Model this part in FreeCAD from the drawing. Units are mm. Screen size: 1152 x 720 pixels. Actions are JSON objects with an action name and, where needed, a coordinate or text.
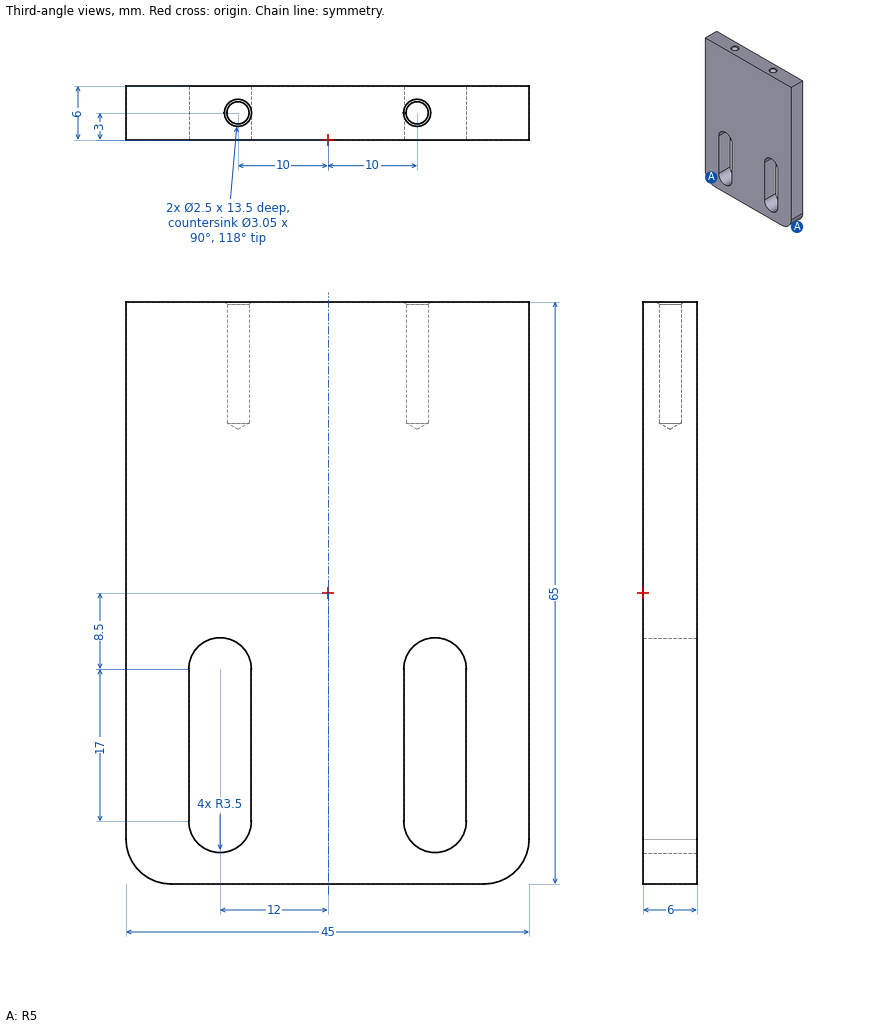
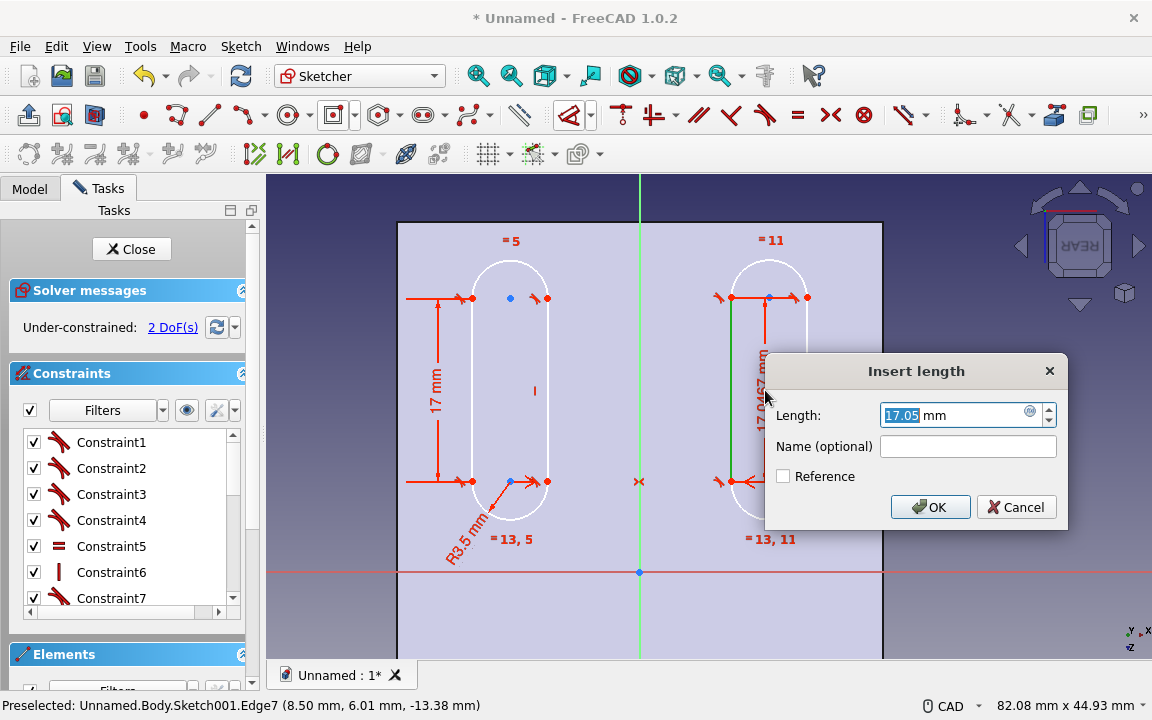
{"action": "type", "text": "17"}
{"action": "key", "text": "Return"}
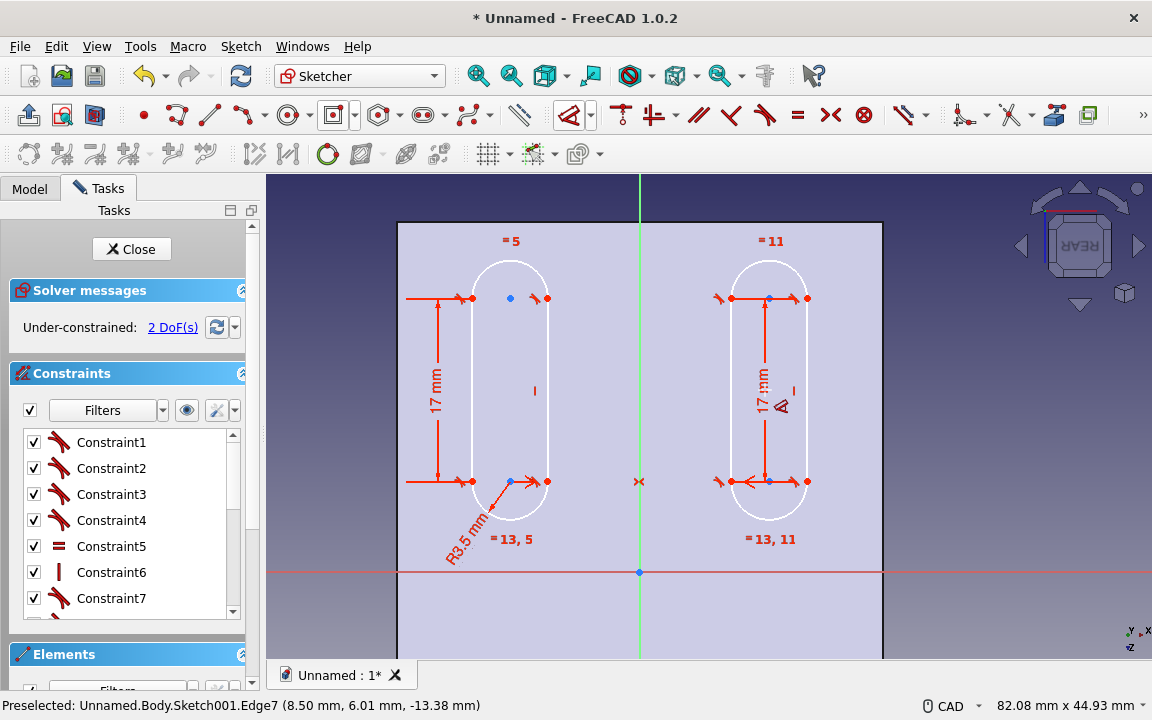
{"action": "left_click", "coordinate": [510, 482]}
{"action": "left_click", "coordinate": [575, 606]}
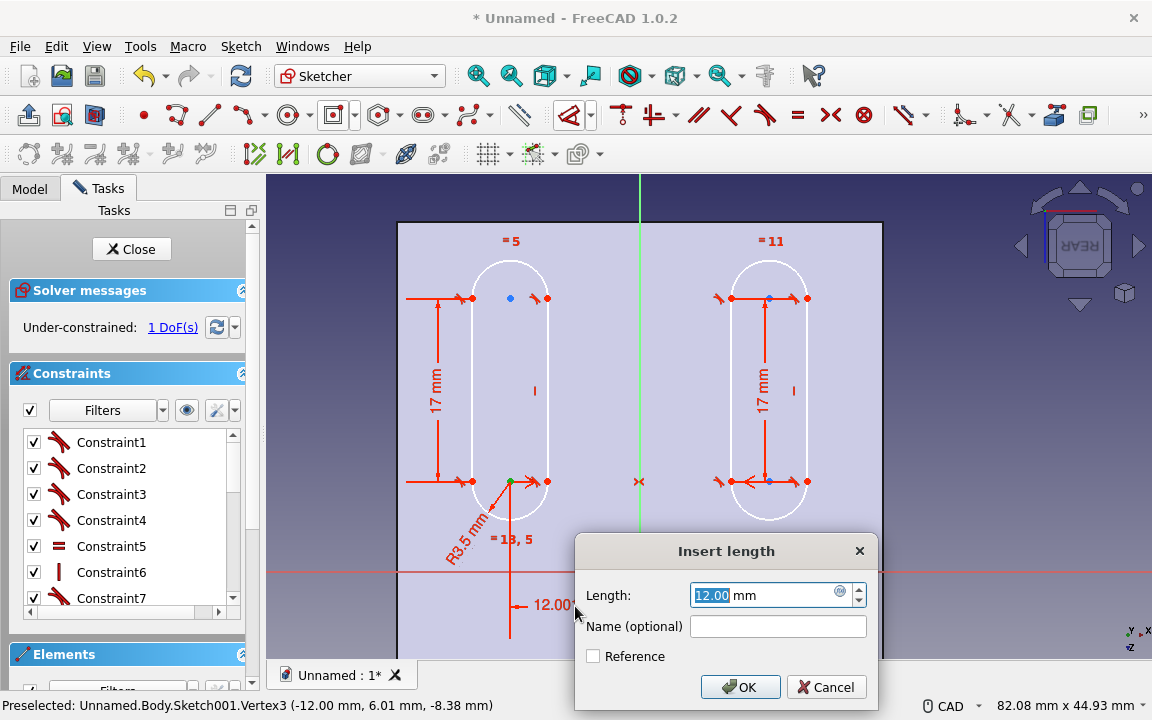
{"action": "type", "text": "12"}
{"action": "key", "text": "Return"}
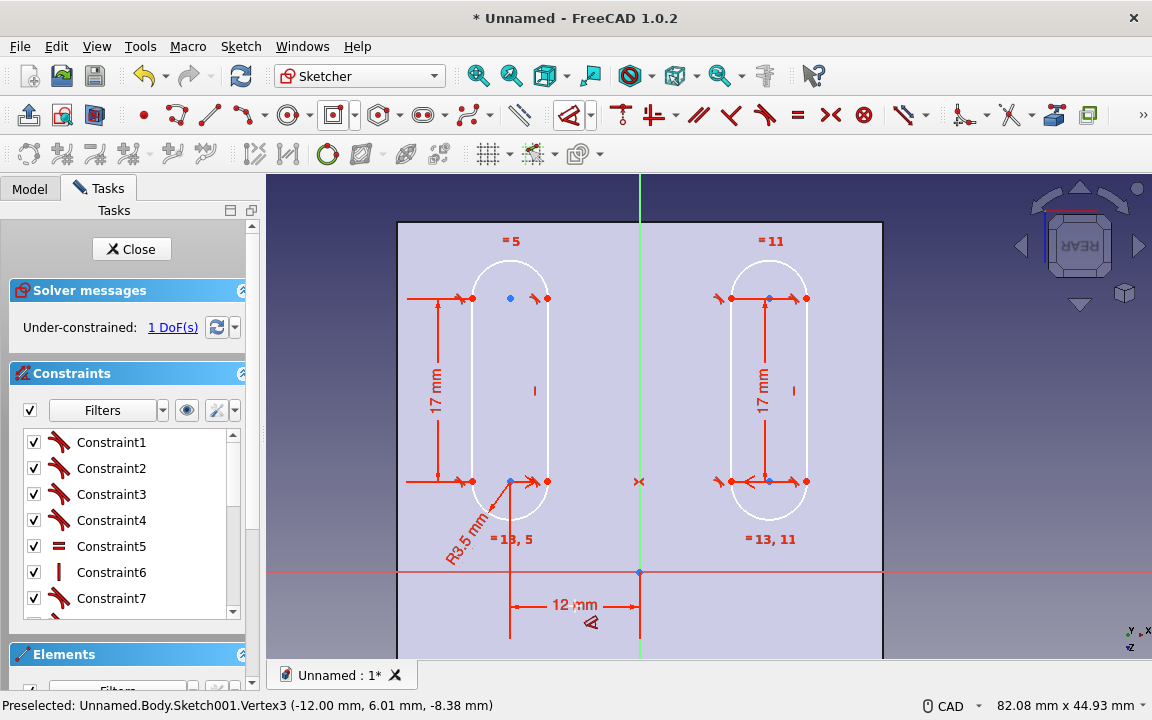
{"action": "left_click", "coordinate": [472, 482]}
{"action": "left_click", "coordinate": [438, 506]}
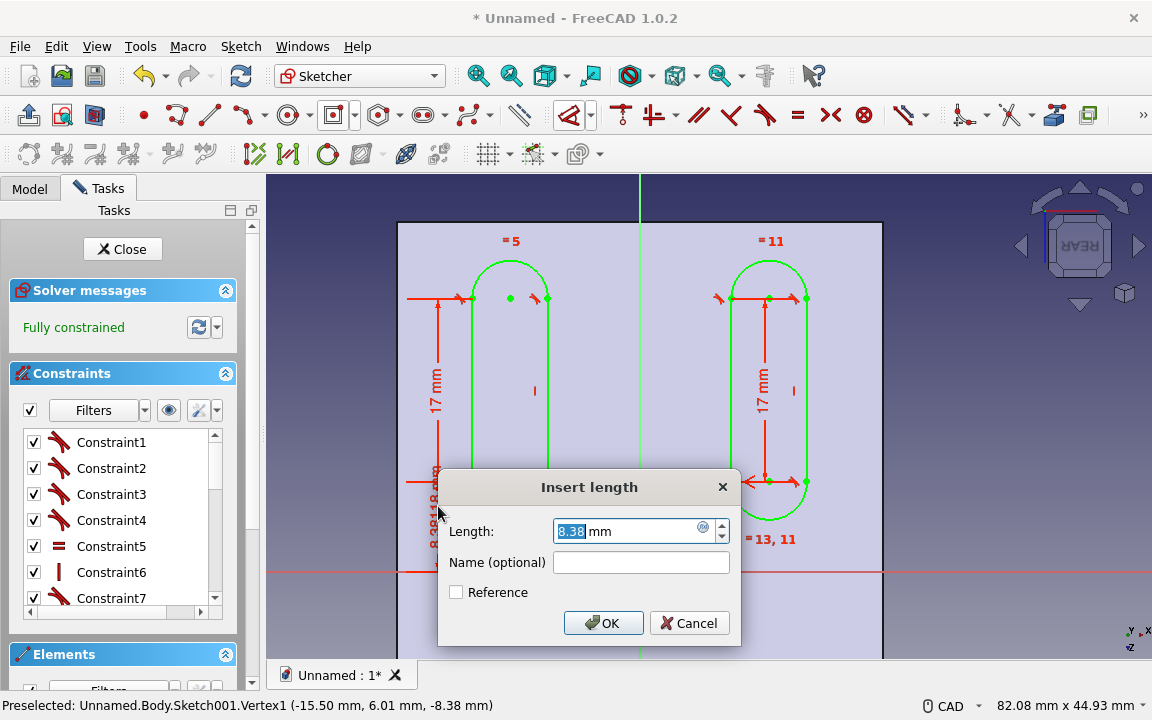
{"action": "type", "text": "8.5"}
{"action": "key", "text": "Return"}
{"action": "key", "text": "Escape"}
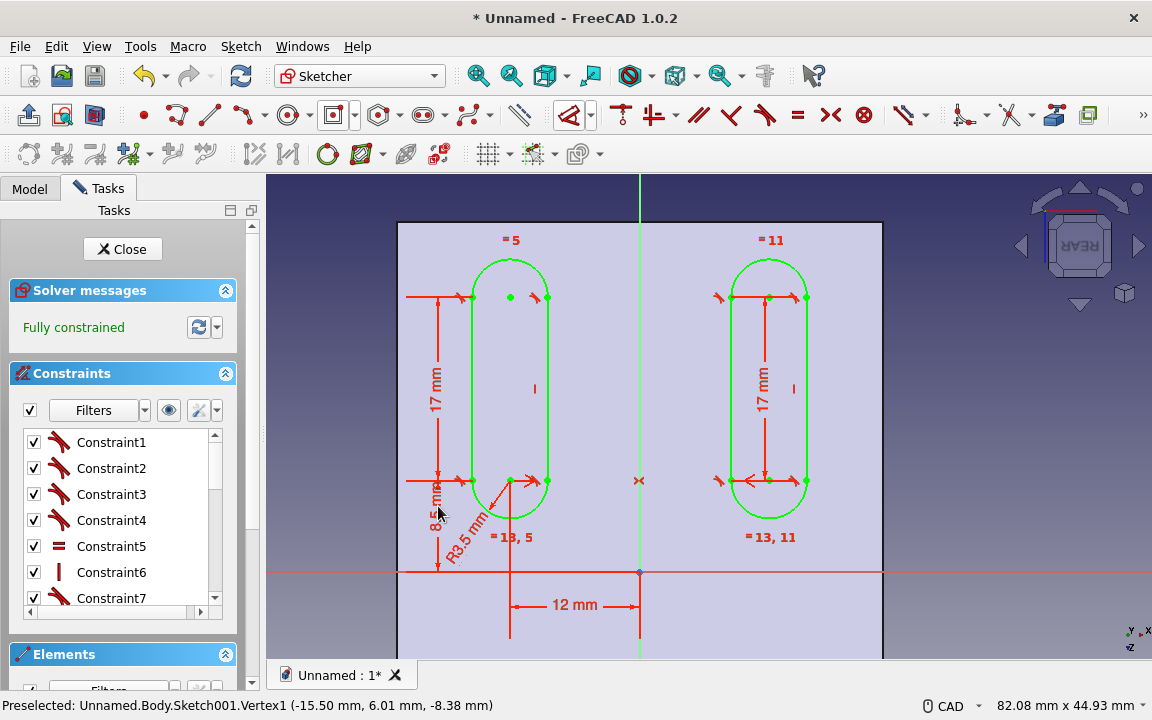
{"action": "left_click", "coordinate": [123, 249]}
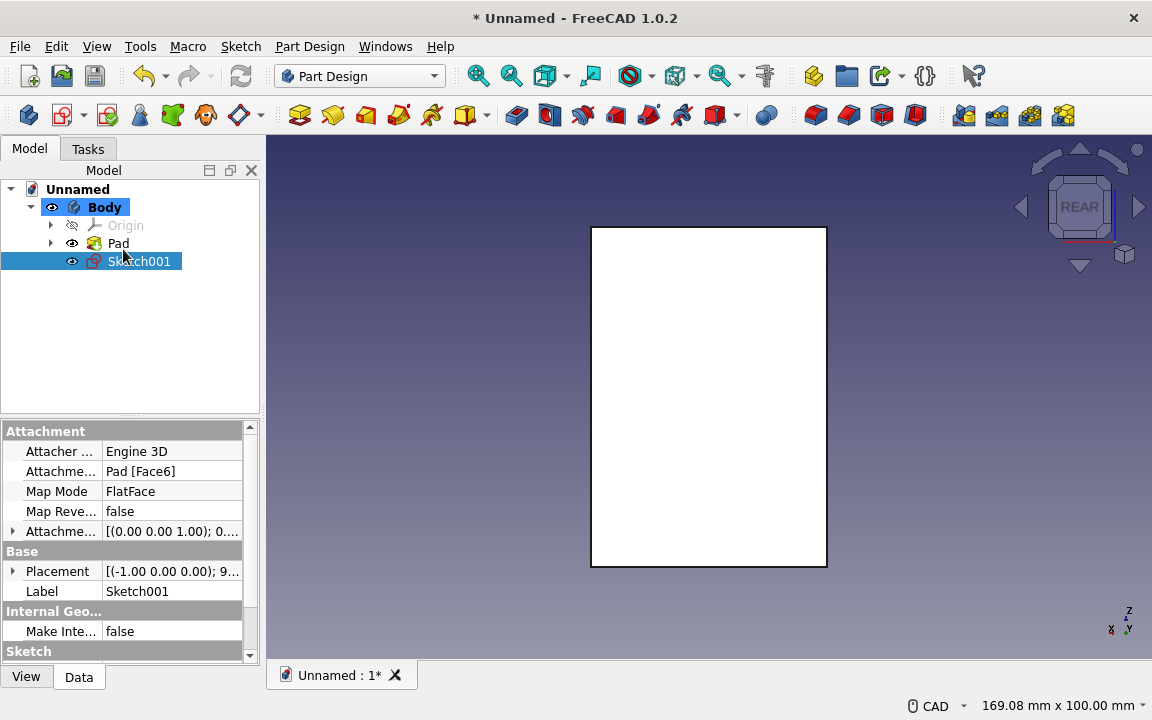
{"action": "left_click", "coordinate": [517, 116]}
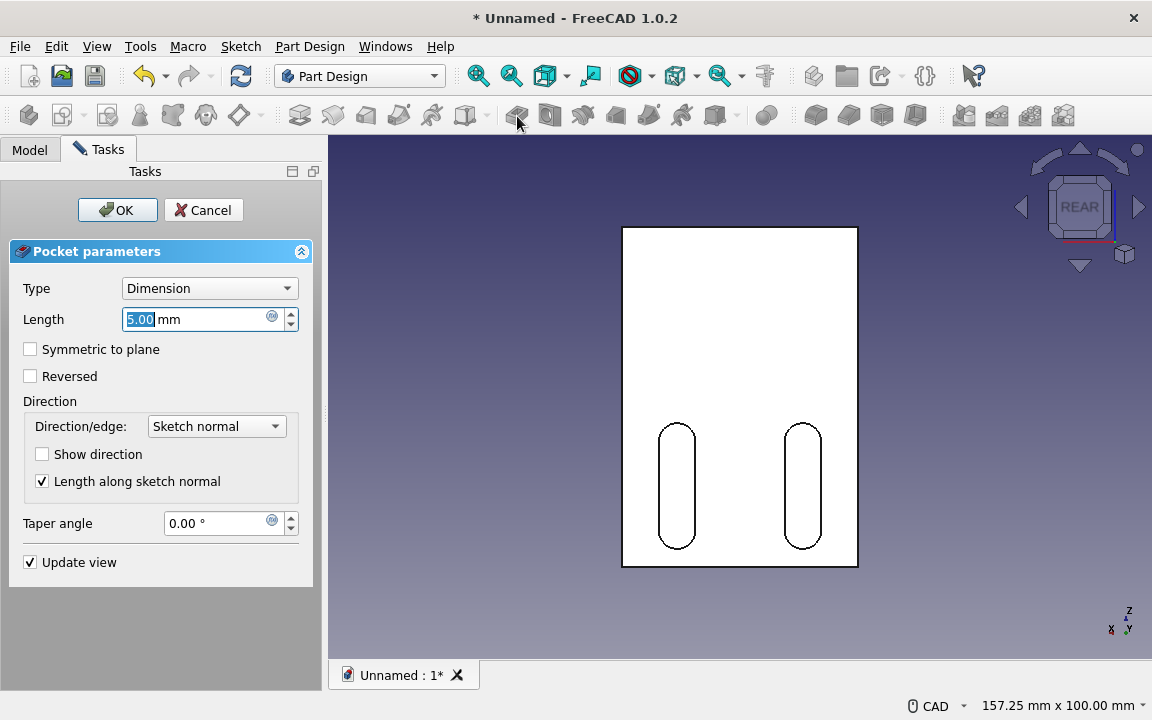
{"action": "type", "text": "6"}
{"action": "key", "text": "Tab"}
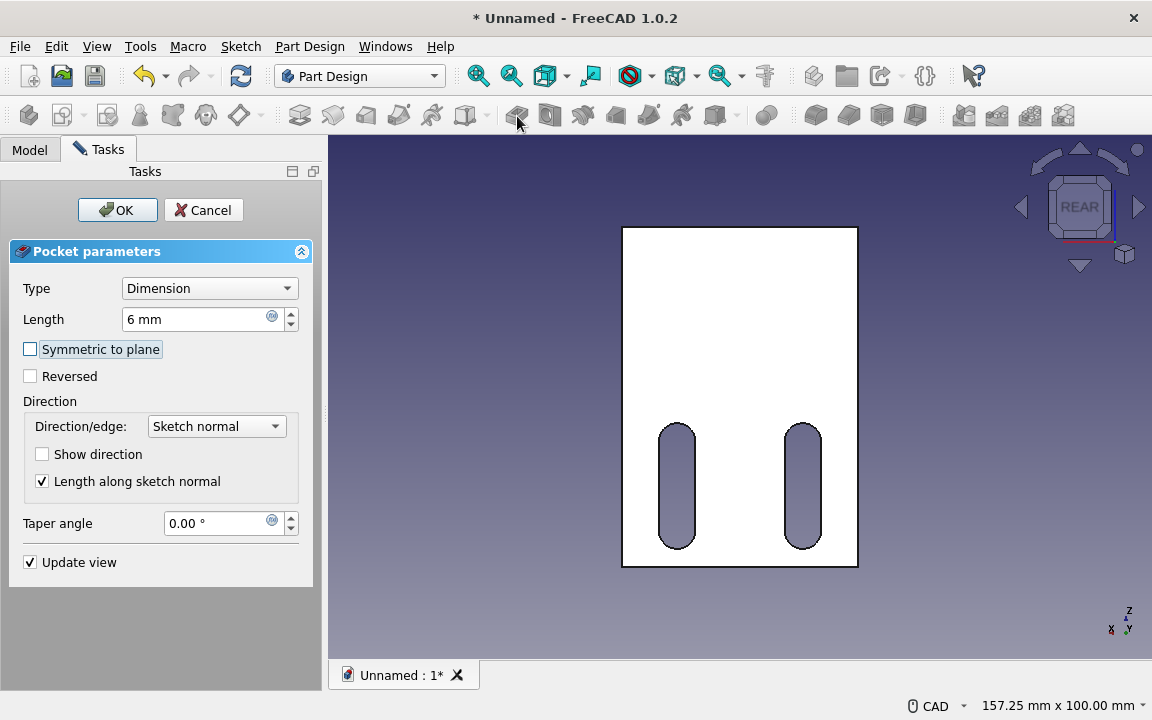
{"action": "left_click", "coordinate": [118, 210]}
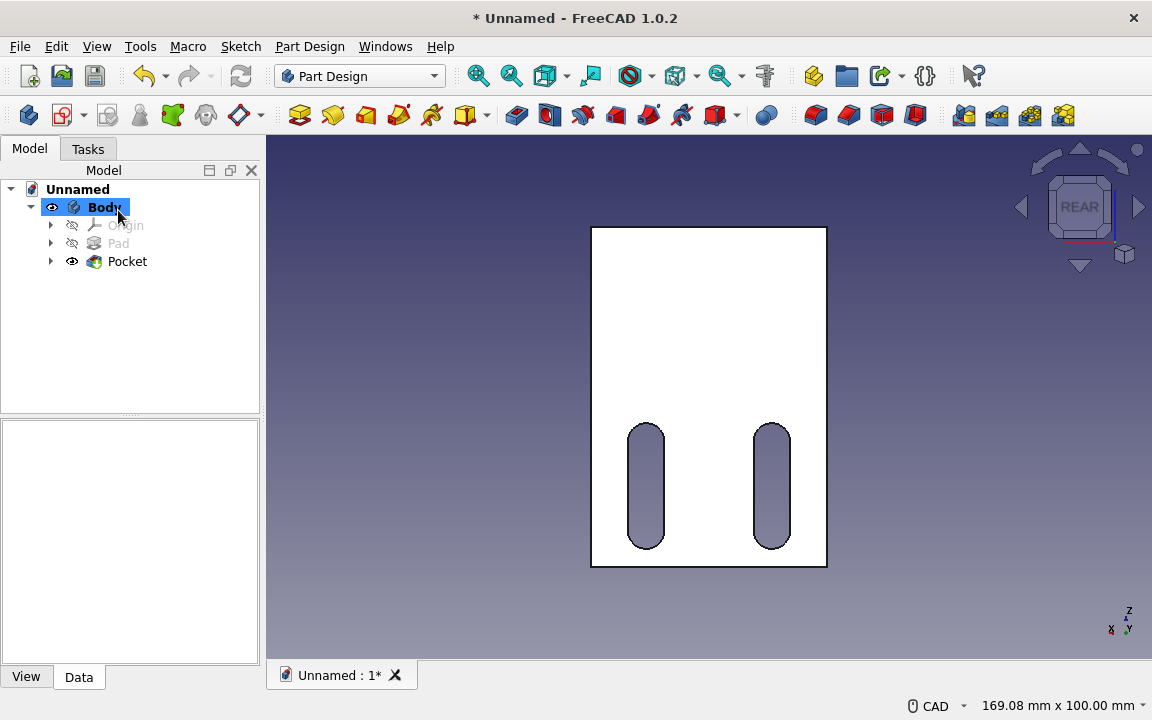
{"action": "key", "text": "0"}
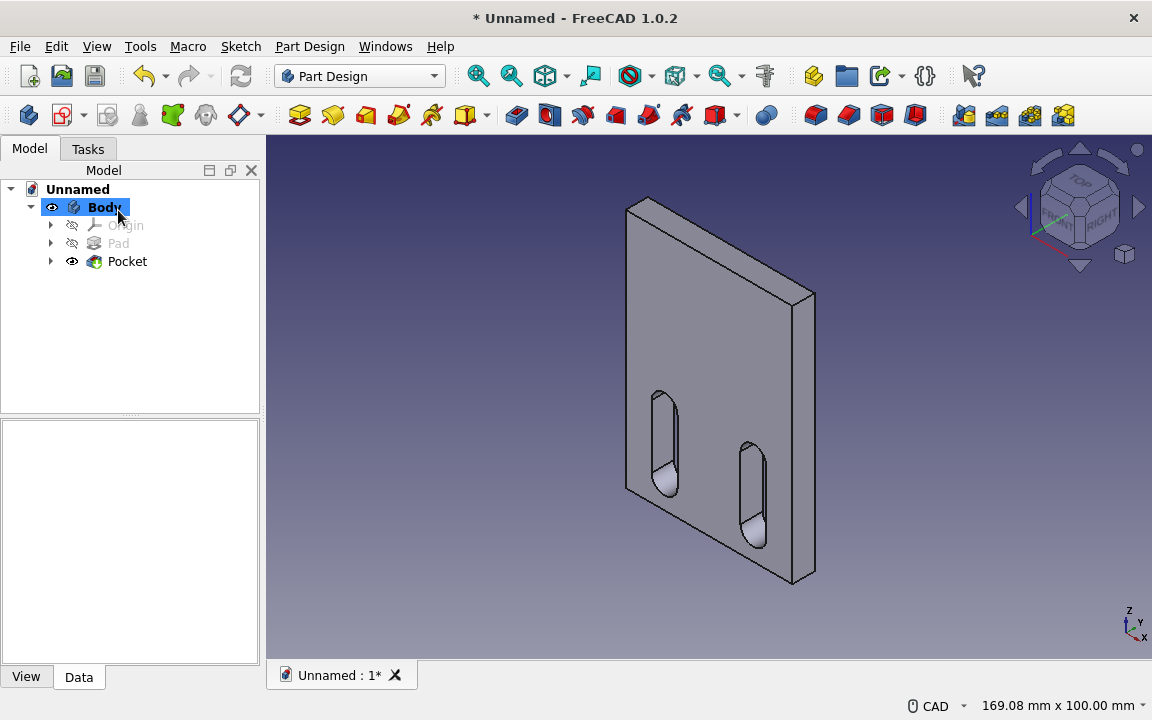
{"action": "key", "text": "2"}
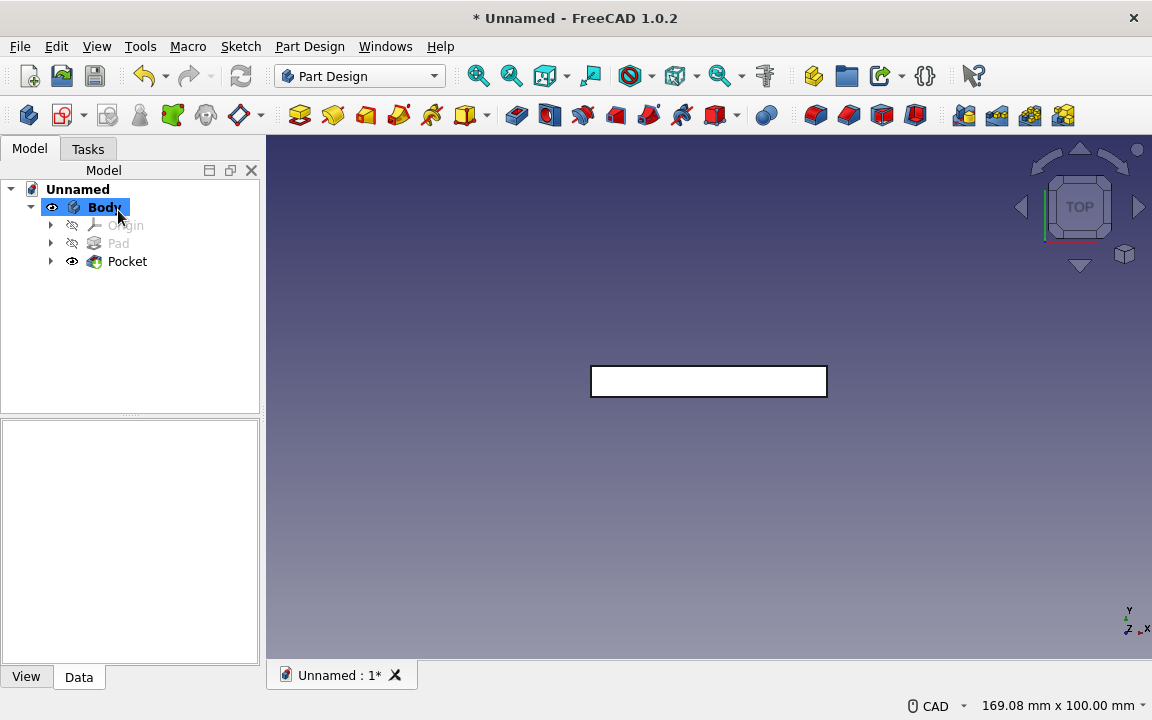
{"action": "key", "text": "v f"}